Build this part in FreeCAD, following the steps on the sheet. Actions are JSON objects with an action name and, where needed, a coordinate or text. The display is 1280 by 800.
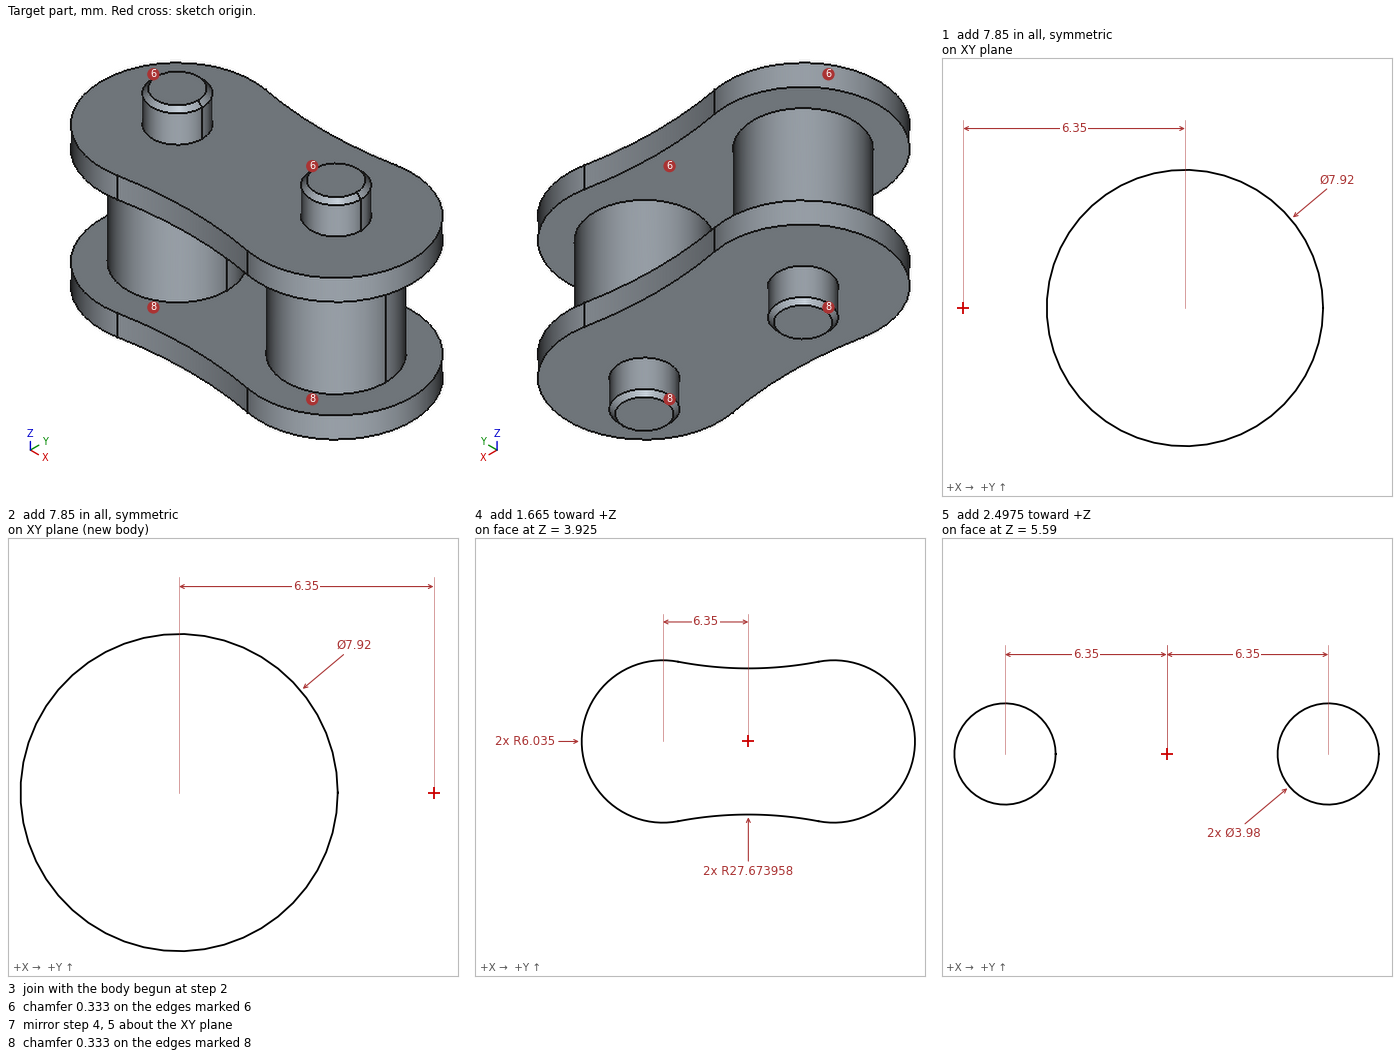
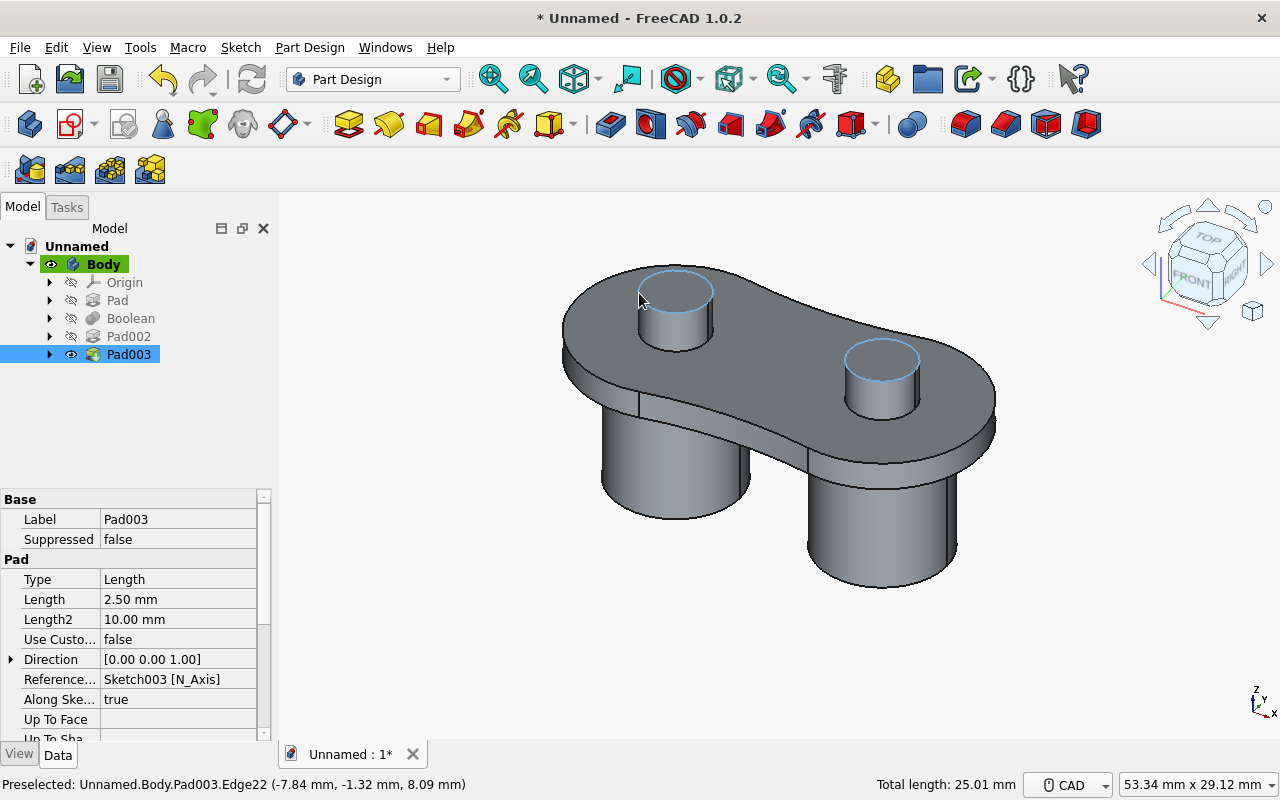
{"action": "left_click", "coordinate": [1006, 124]}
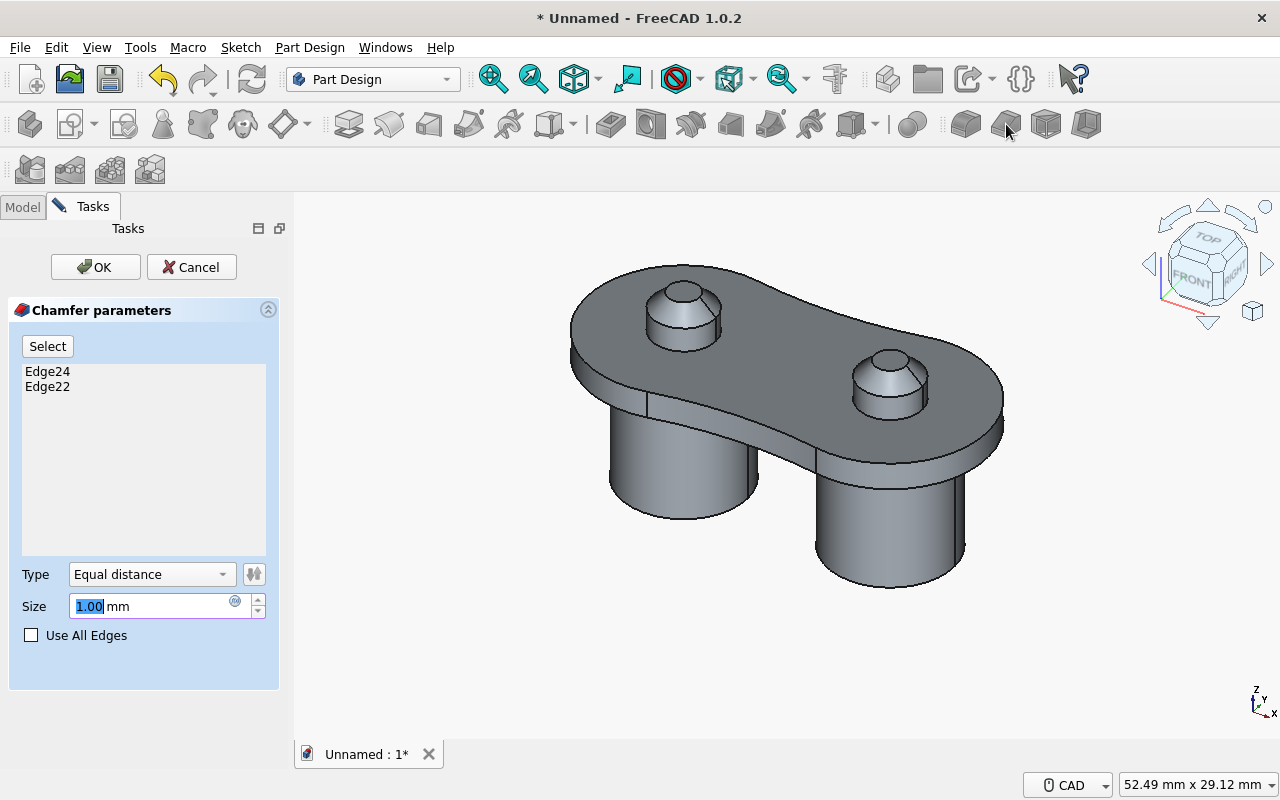
{"action": "type", "text": "0.333"}
{"action": "key", "text": "Tab"}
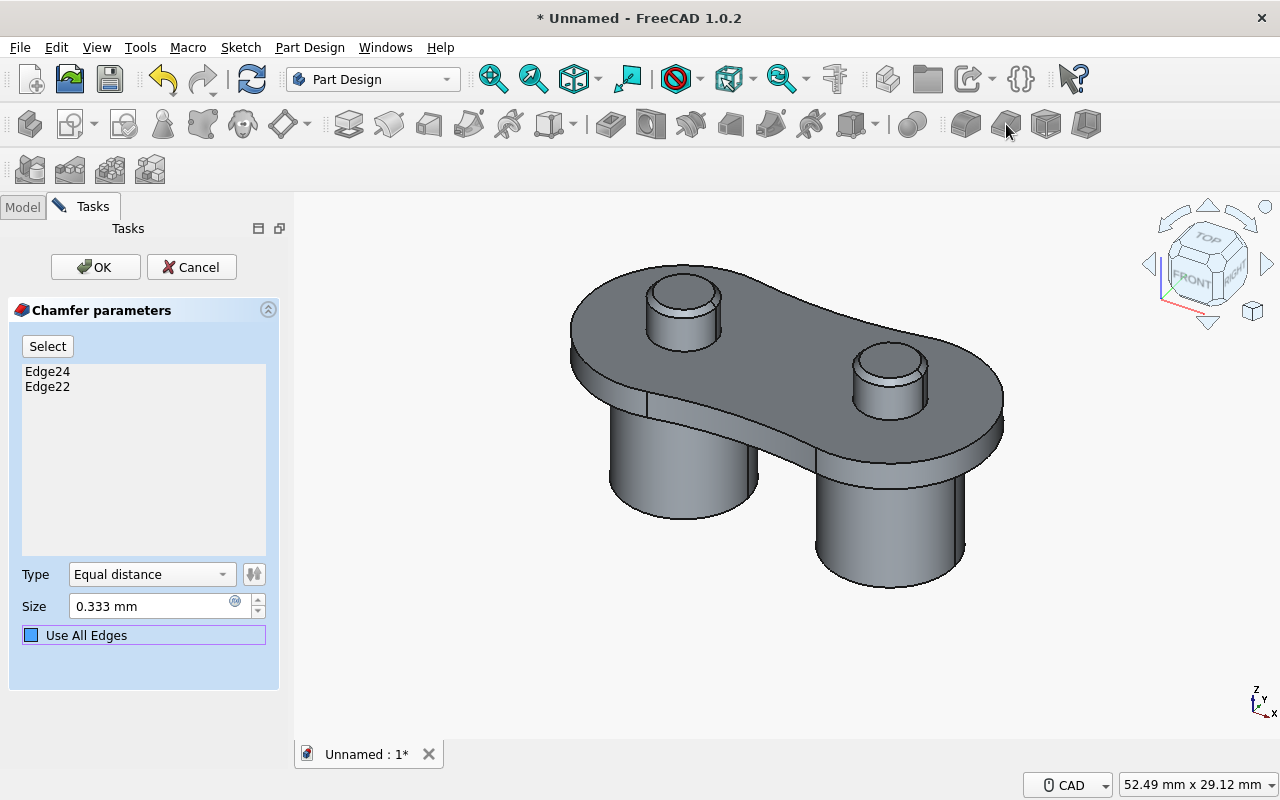
{"action": "left_click", "coordinate": [96, 267]}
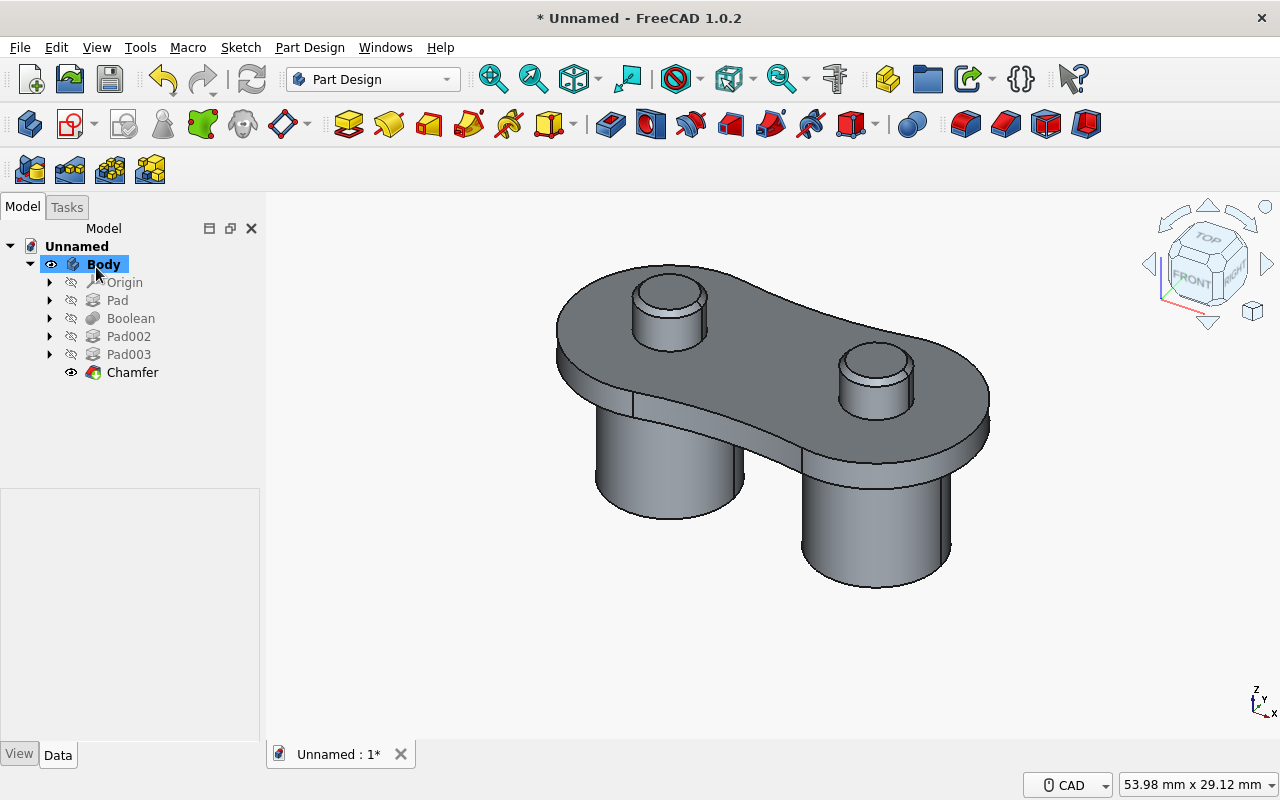
{"action": "left_click", "coordinate": [116, 336]}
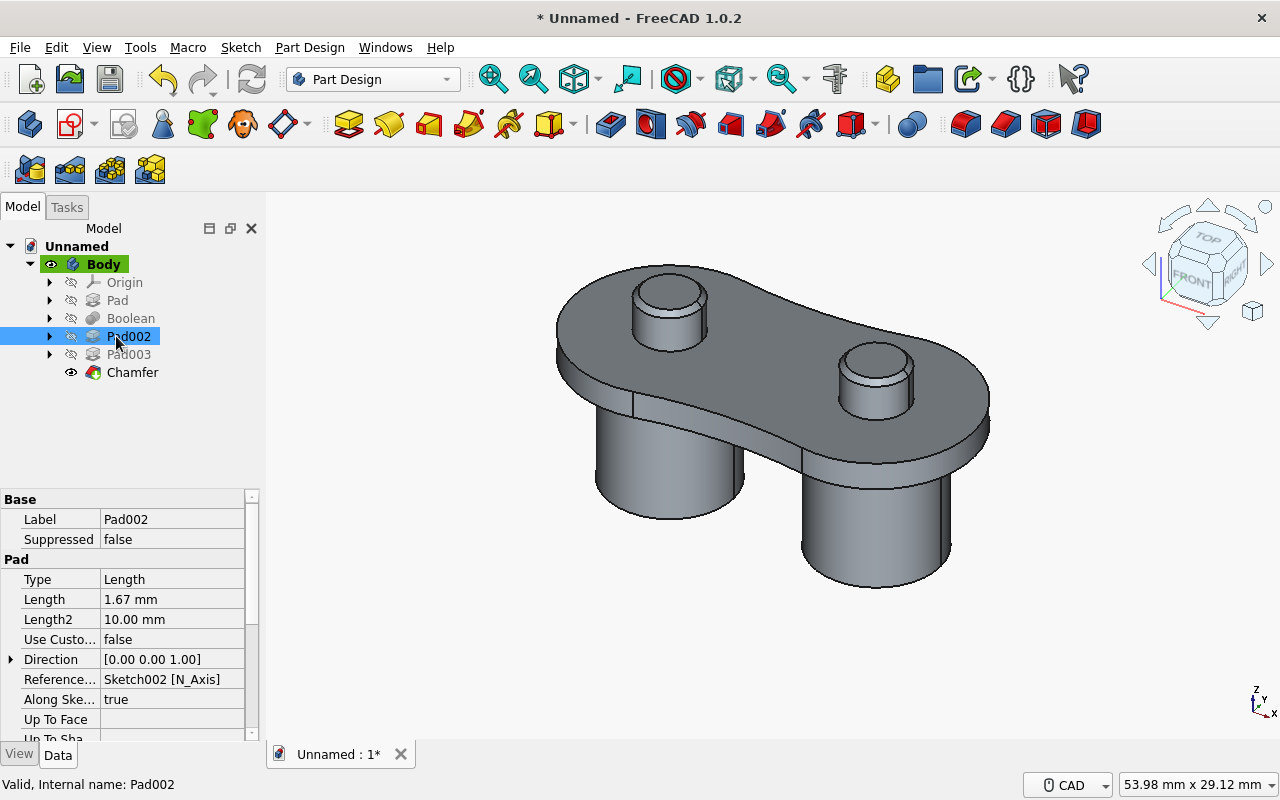
{"action": "left_click", "coordinate": [116, 354], "text": "ctrl"}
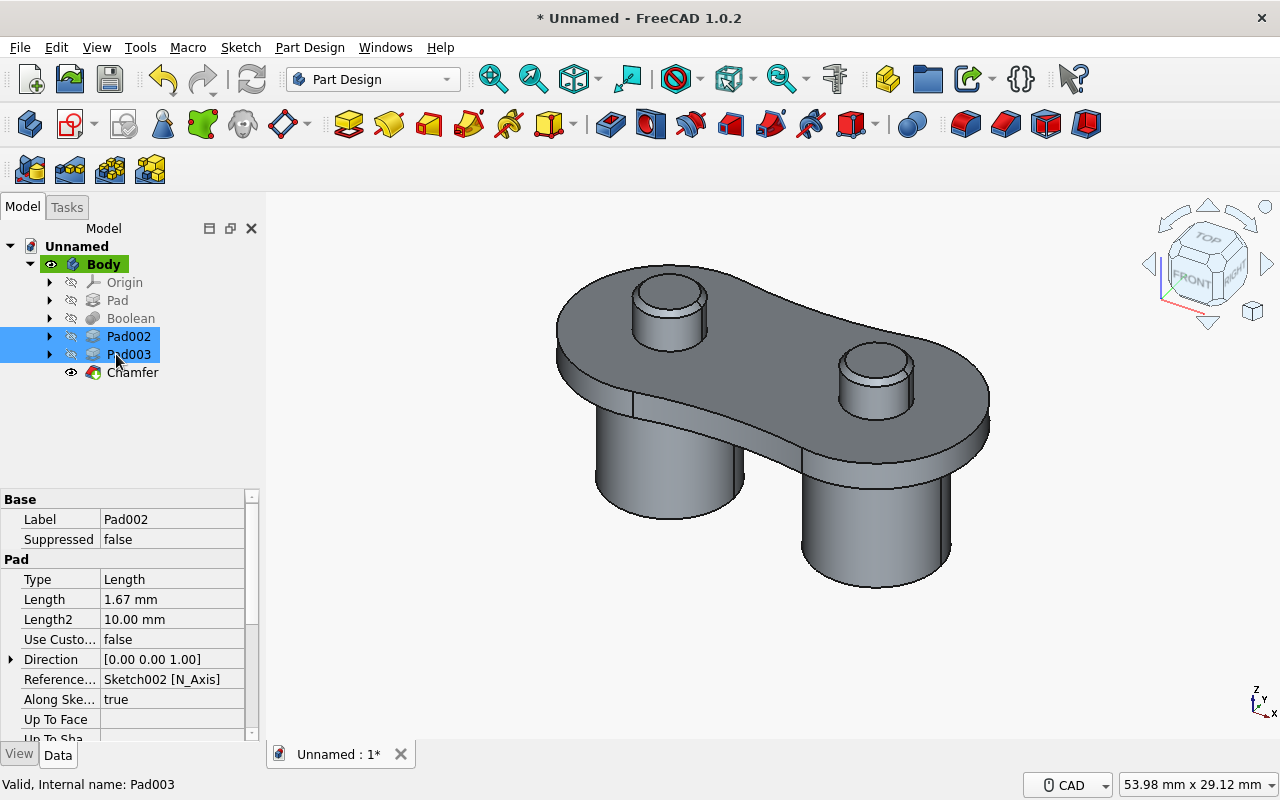
{"action": "left_click", "coordinate": [30, 170]}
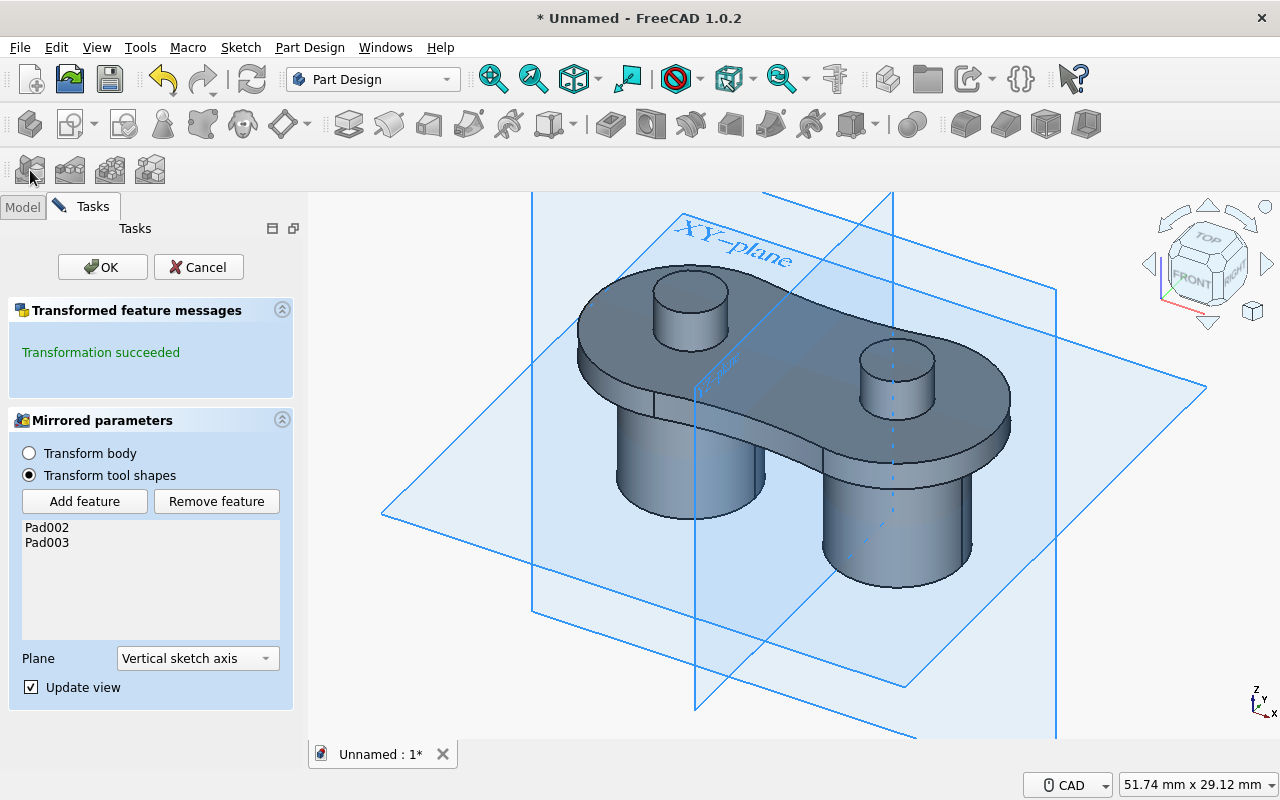
{"action": "left_click", "coordinate": [198, 658]}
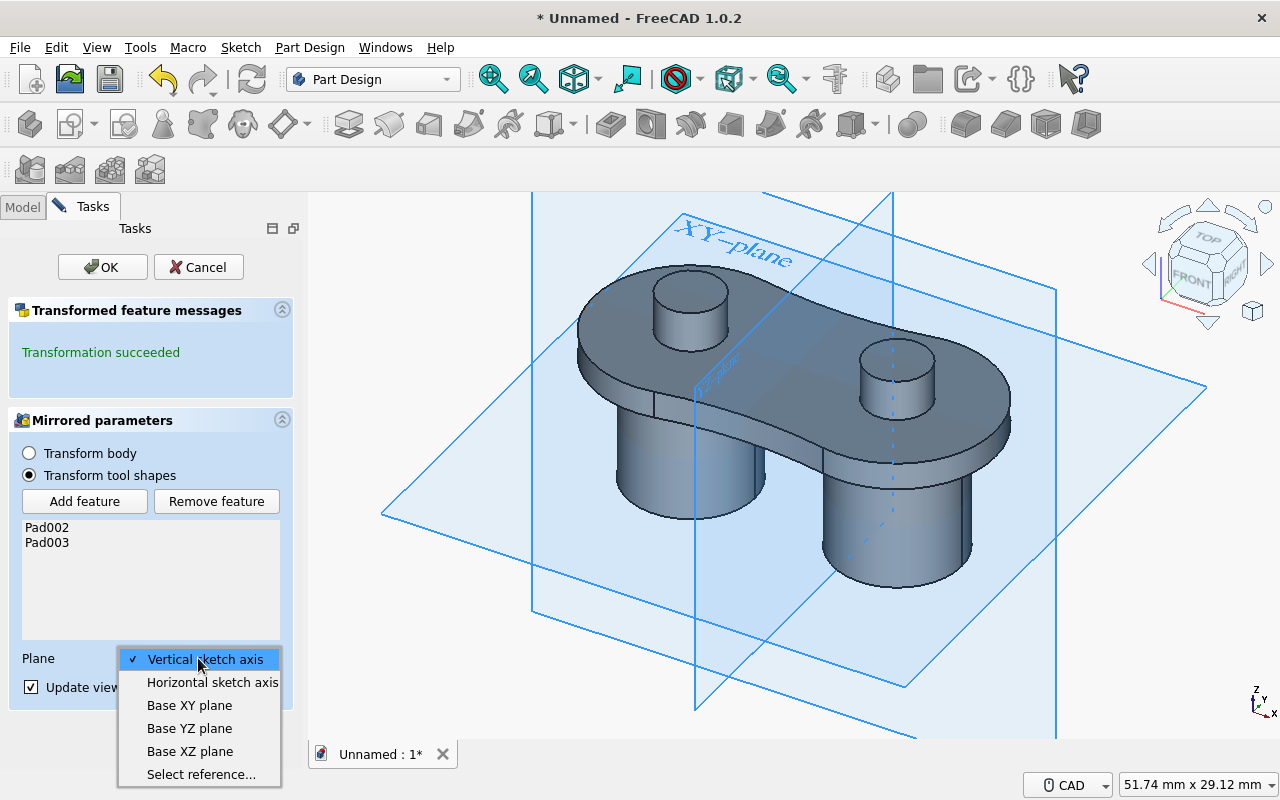
{"action": "left_click", "coordinate": [198, 706]}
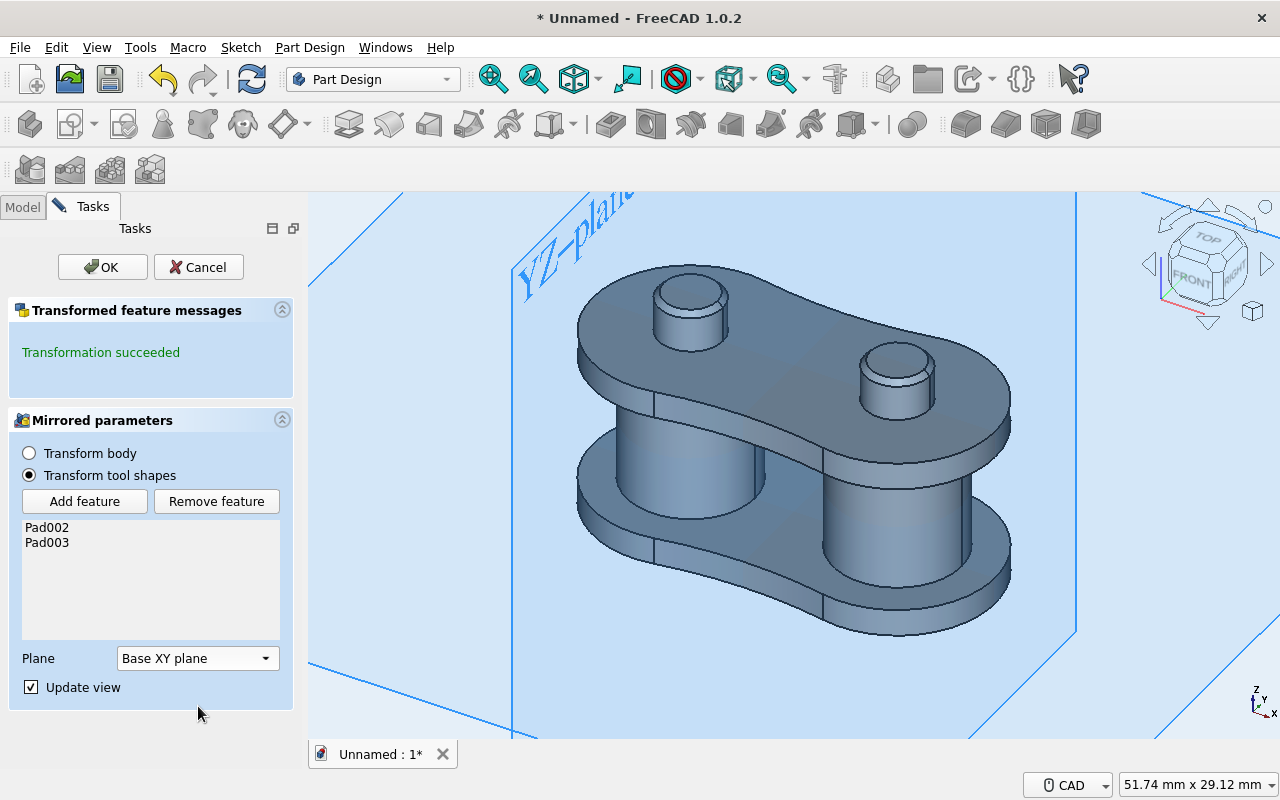
{"action": "left_click", "coordinate": [103, 267]}